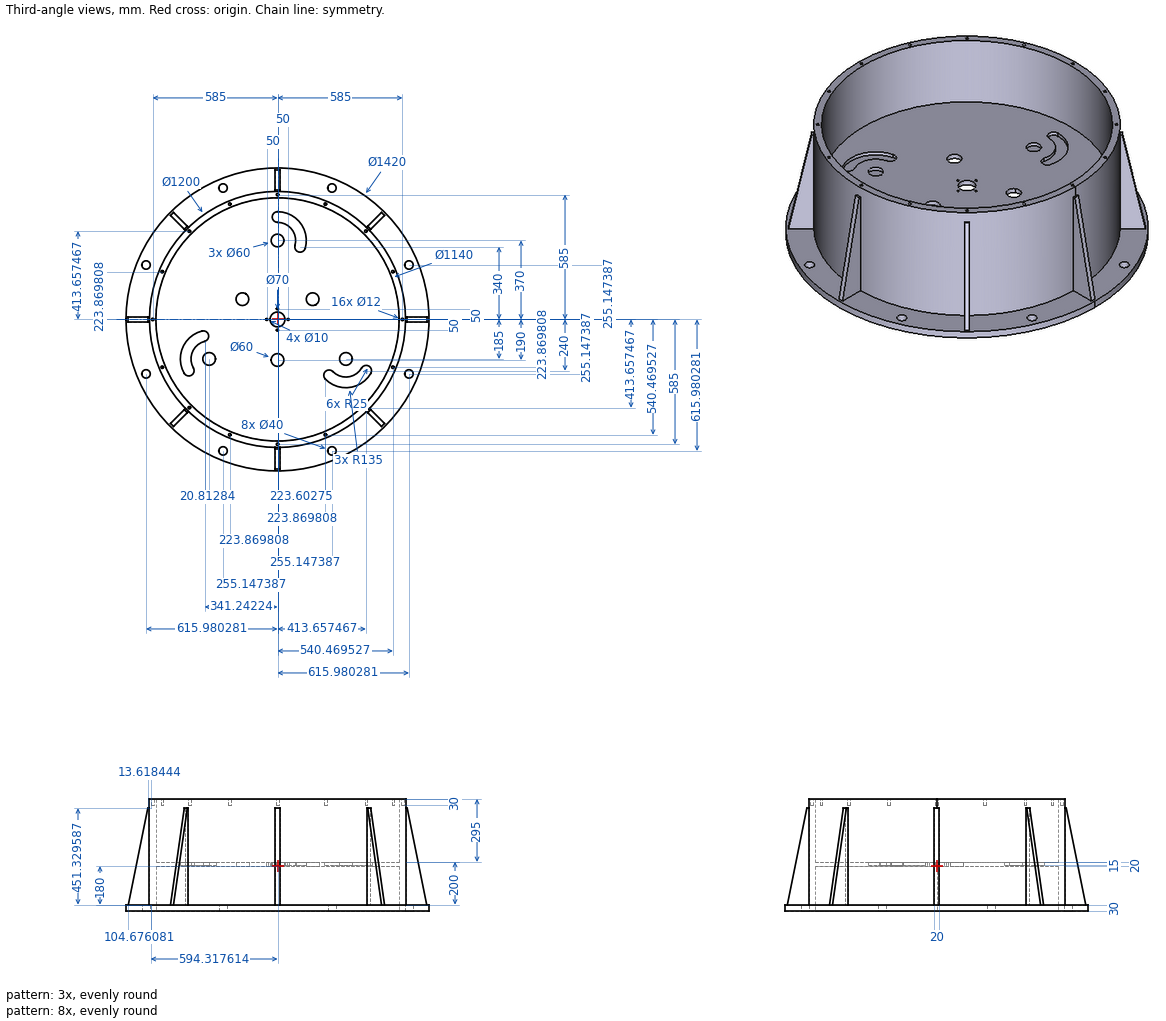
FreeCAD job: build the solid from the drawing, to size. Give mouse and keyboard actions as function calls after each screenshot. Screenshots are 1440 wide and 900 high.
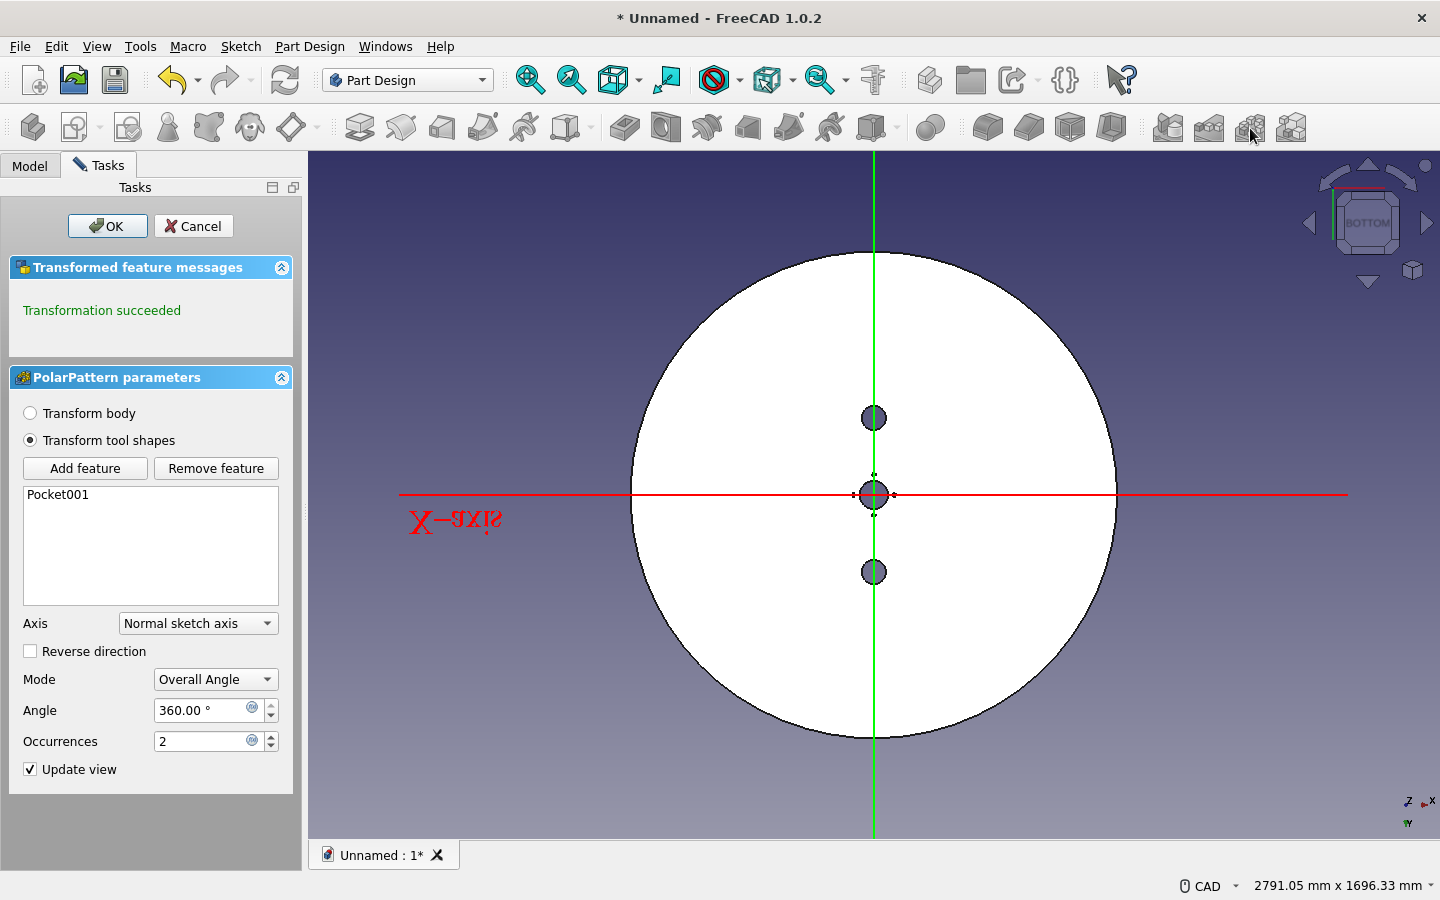
click(199, 624)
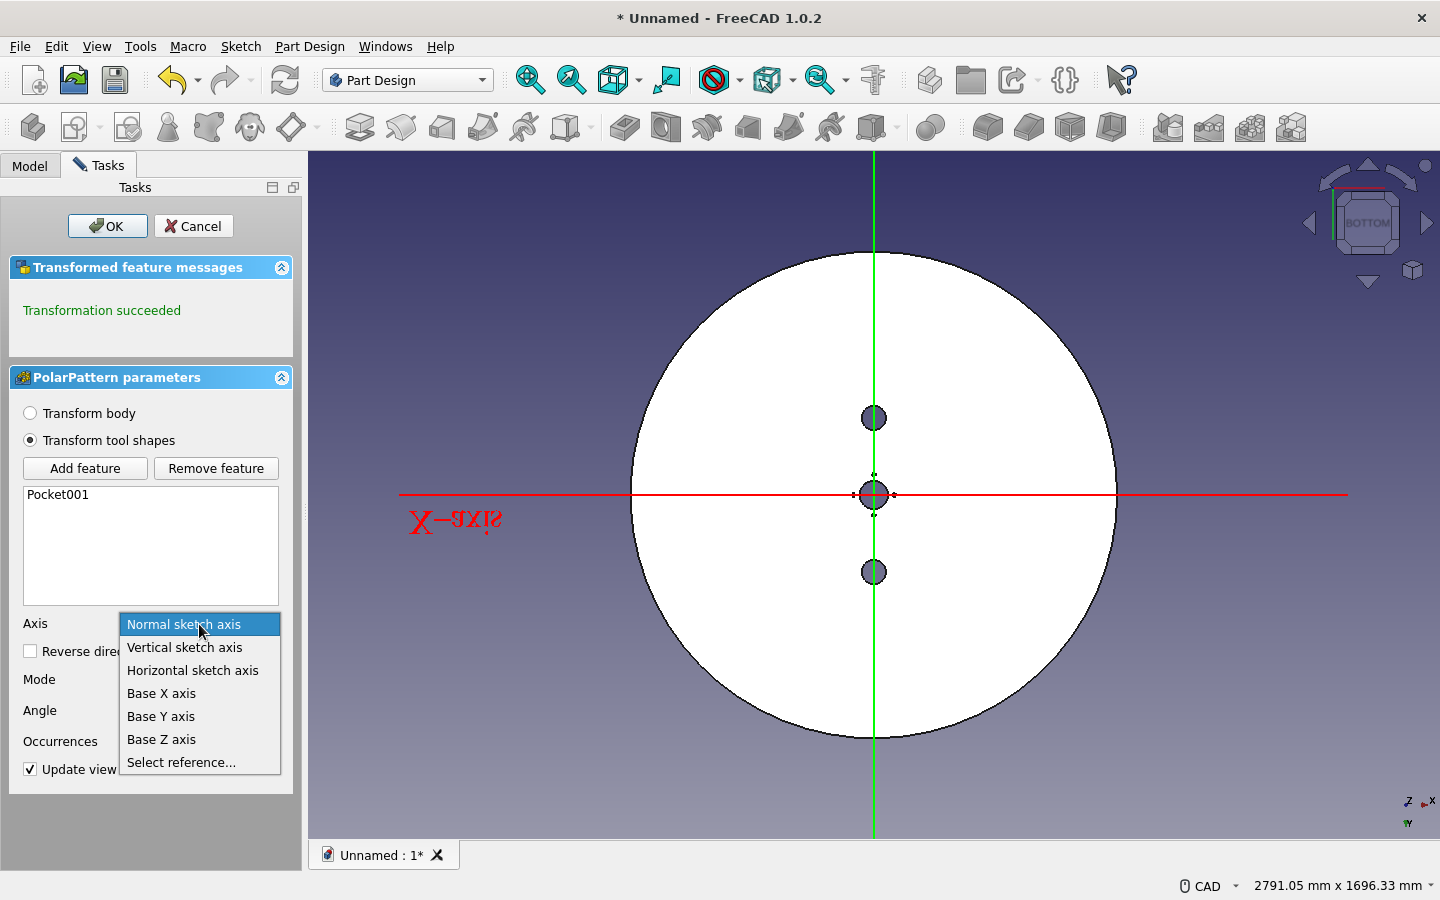
click(198, 740)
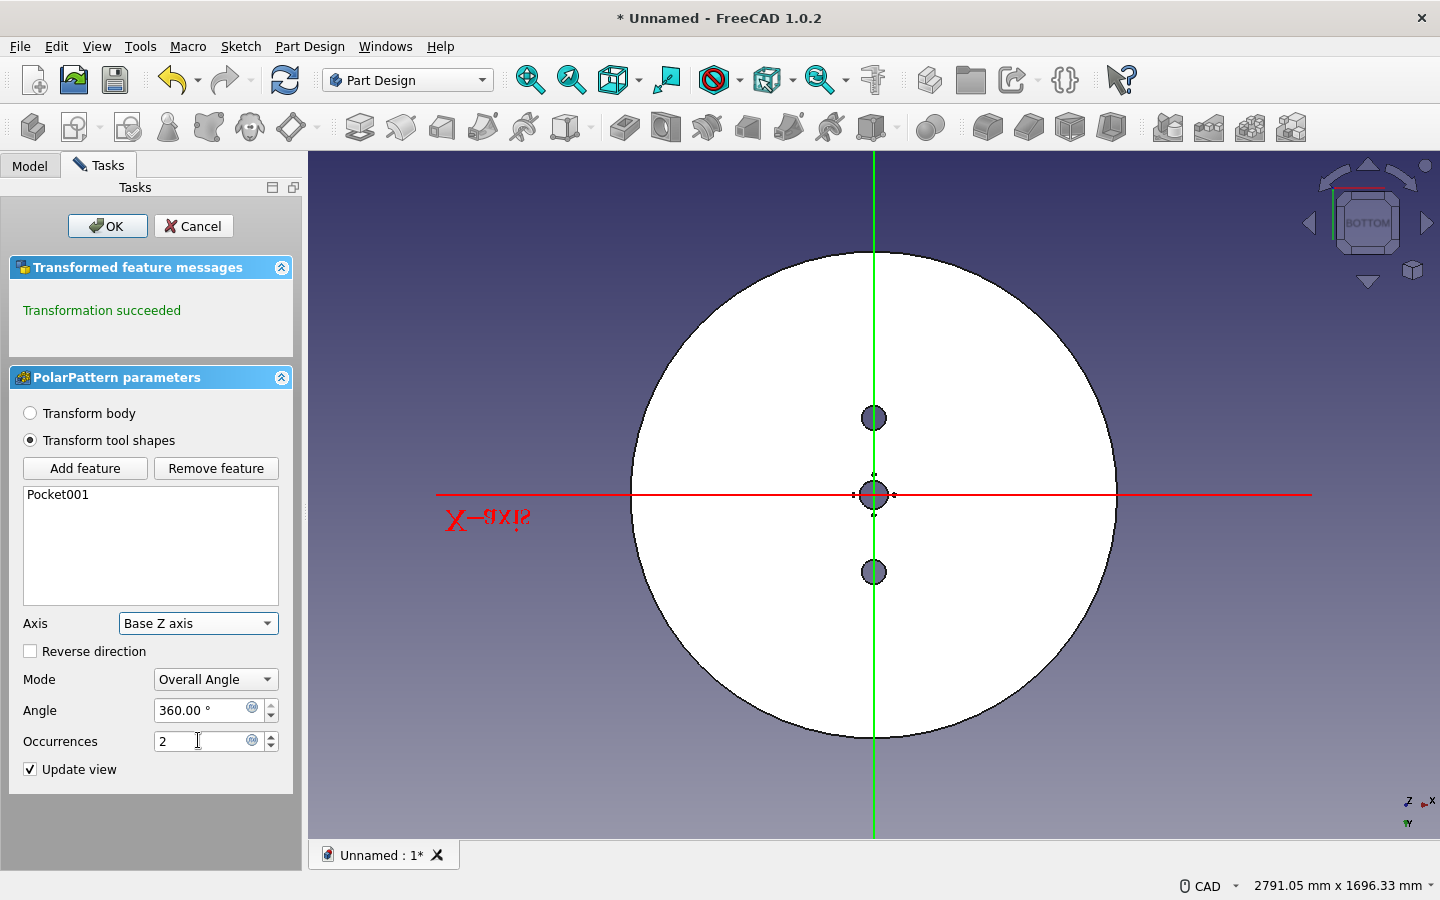
triple_click(210, 742)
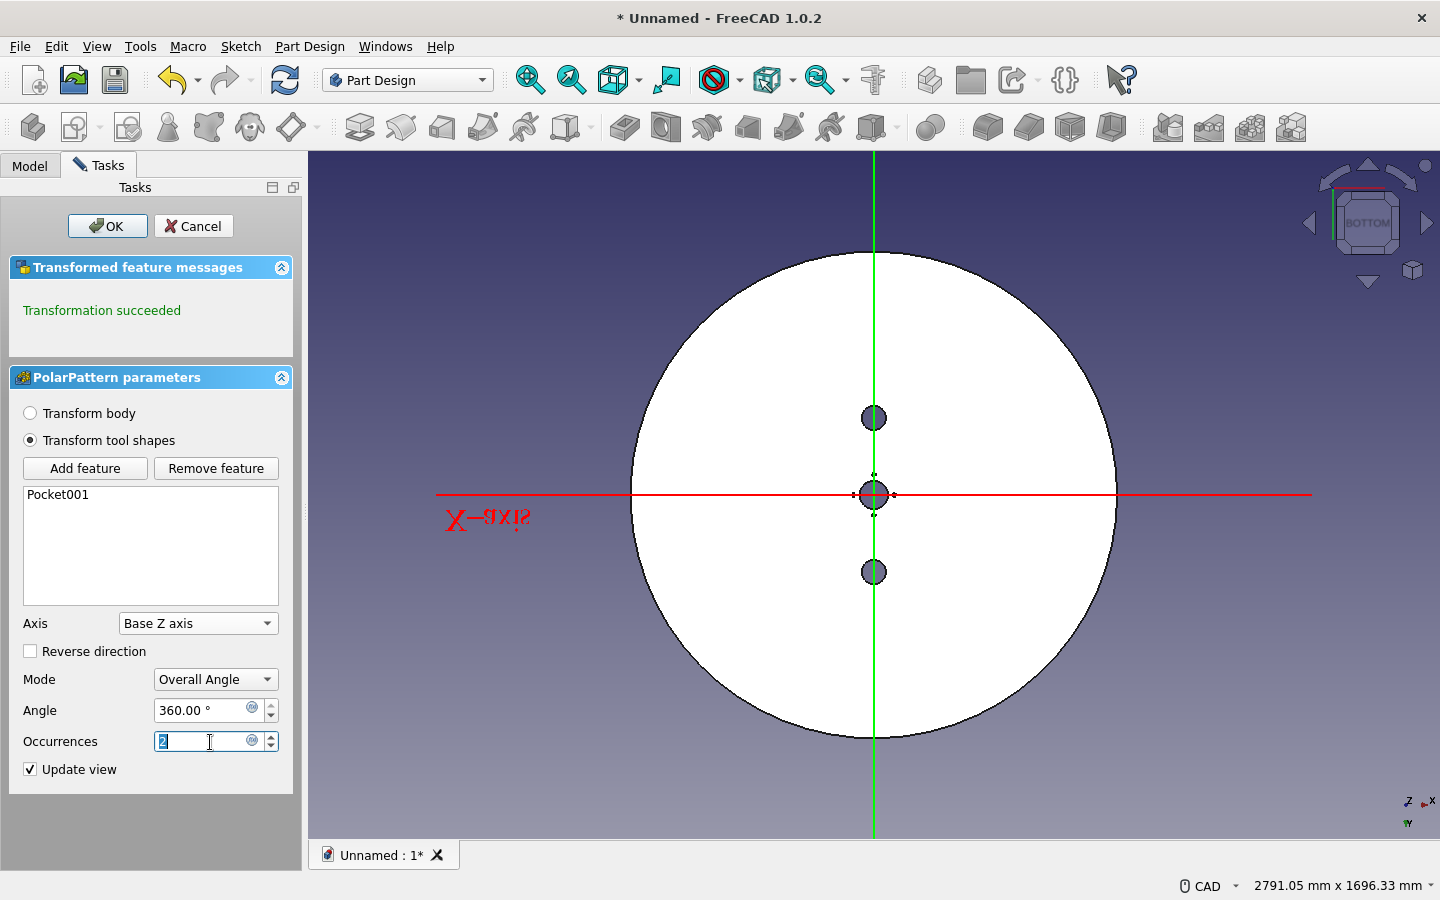
text(3)
key(Tab)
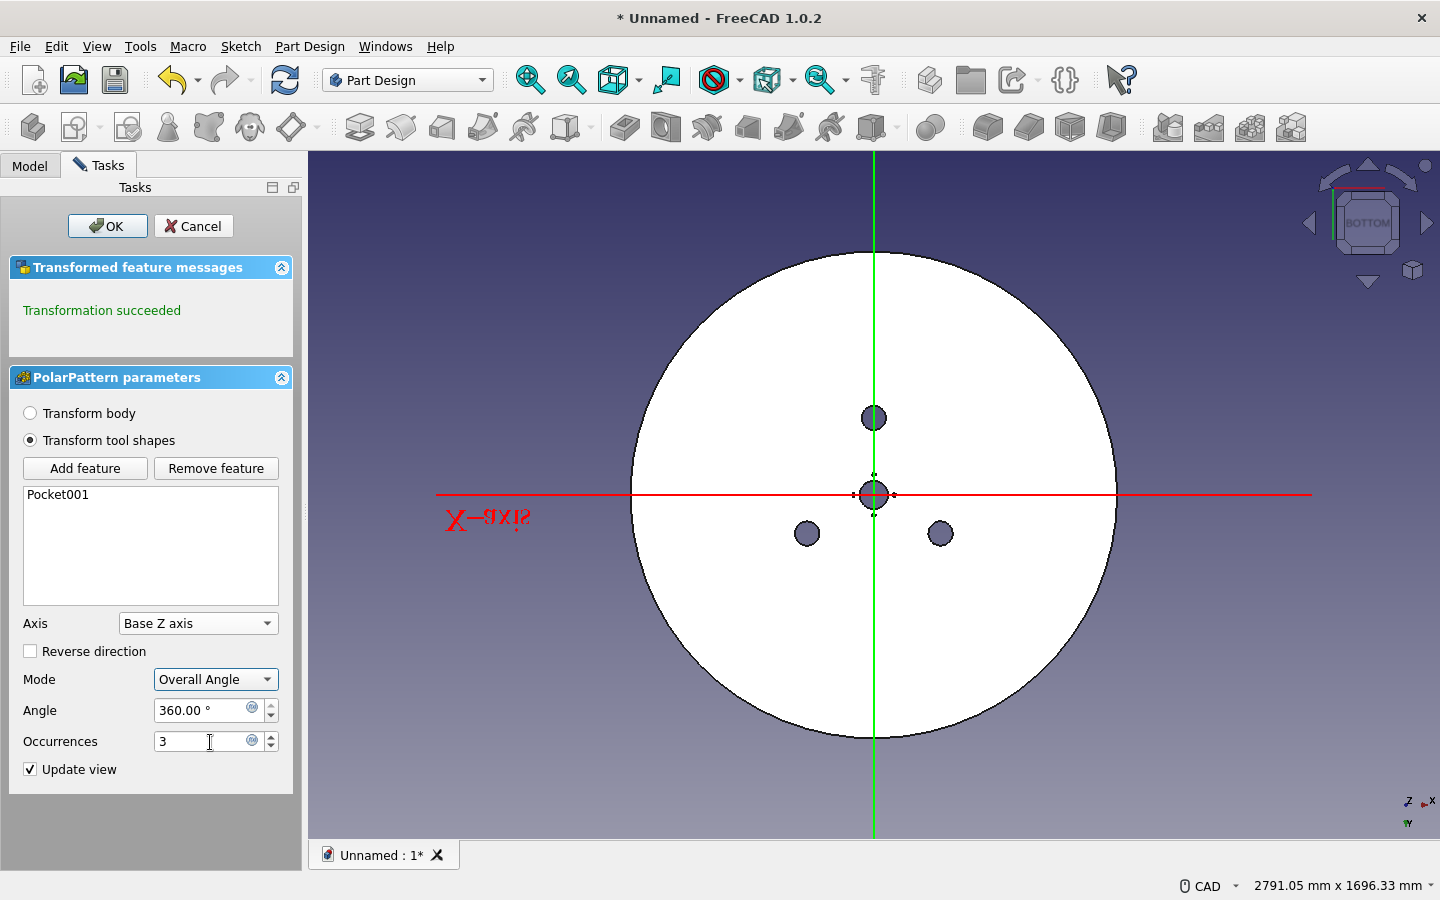
click(108, 226)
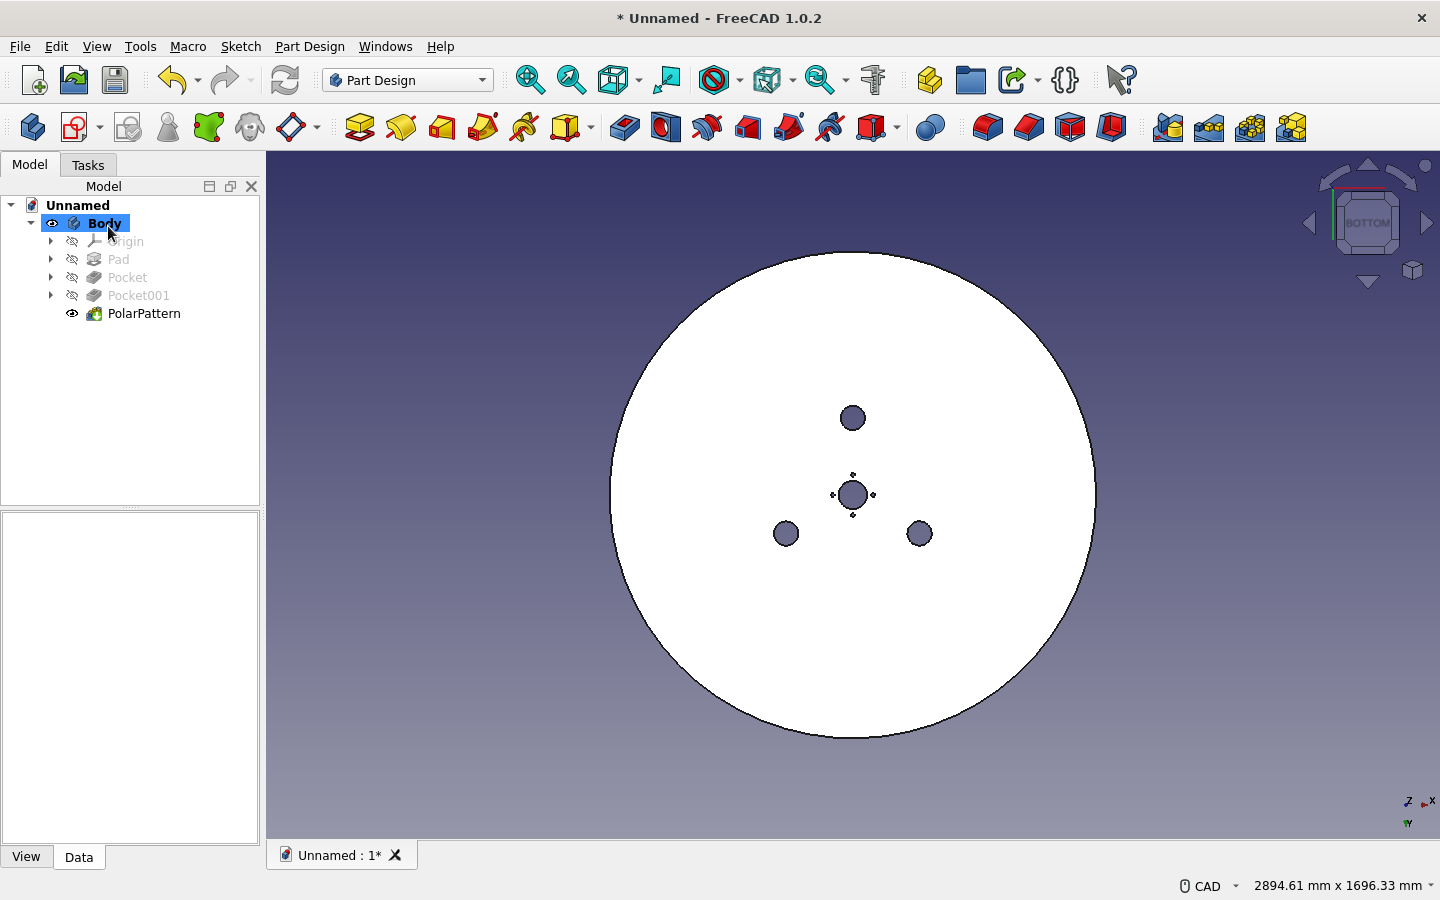
click(51, 241)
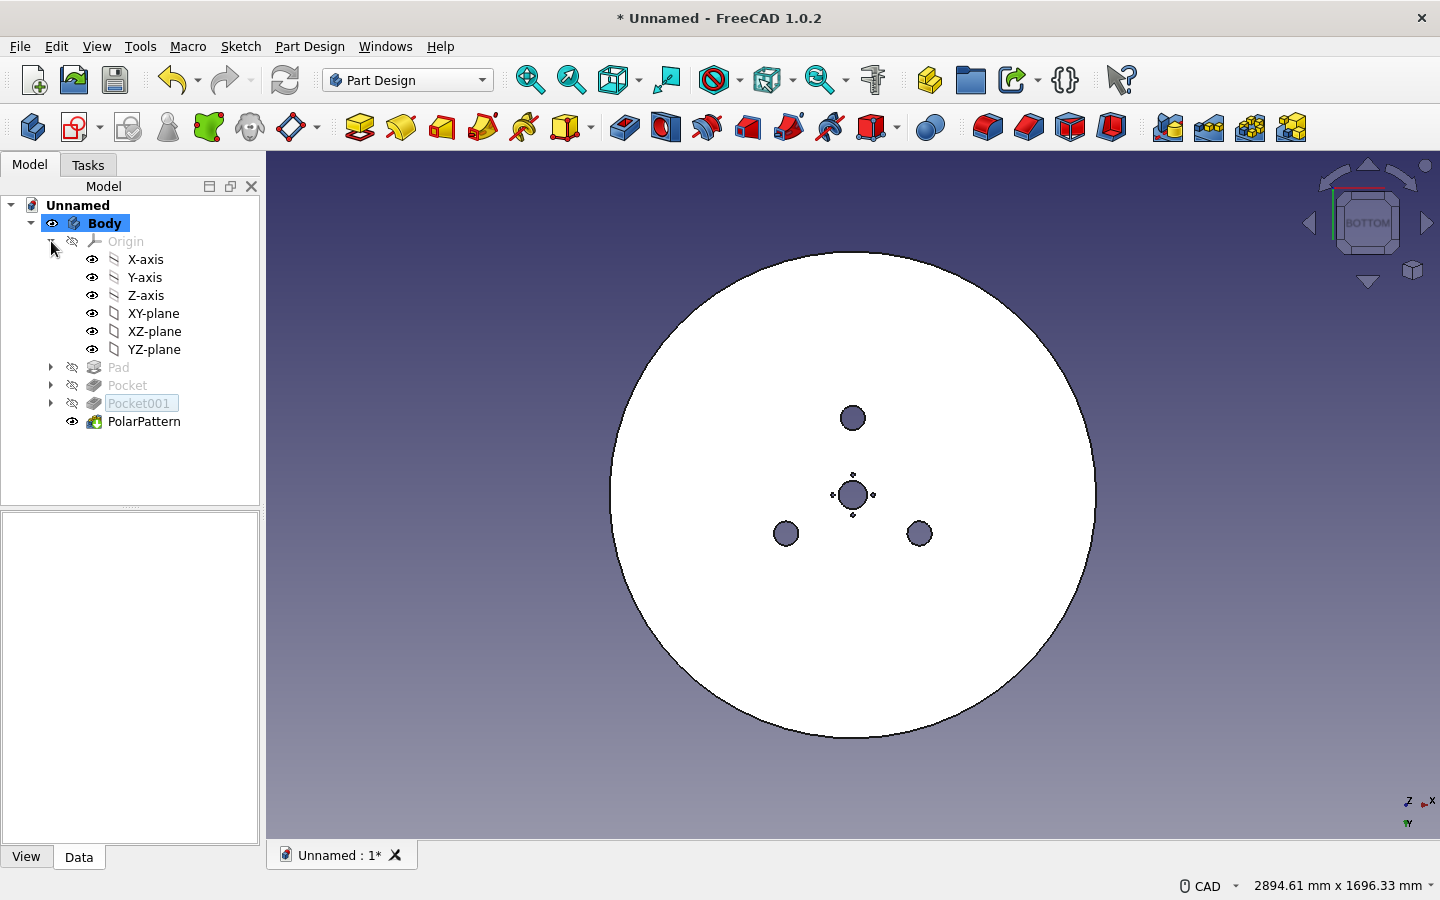
click(137, 313)